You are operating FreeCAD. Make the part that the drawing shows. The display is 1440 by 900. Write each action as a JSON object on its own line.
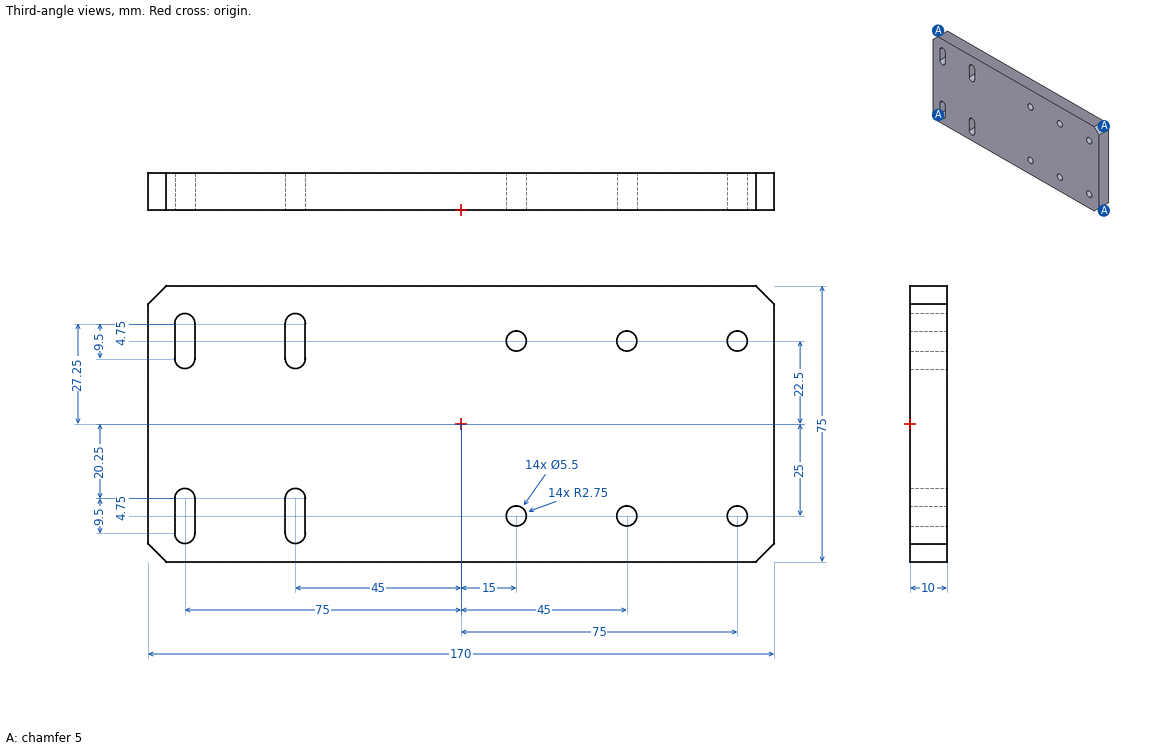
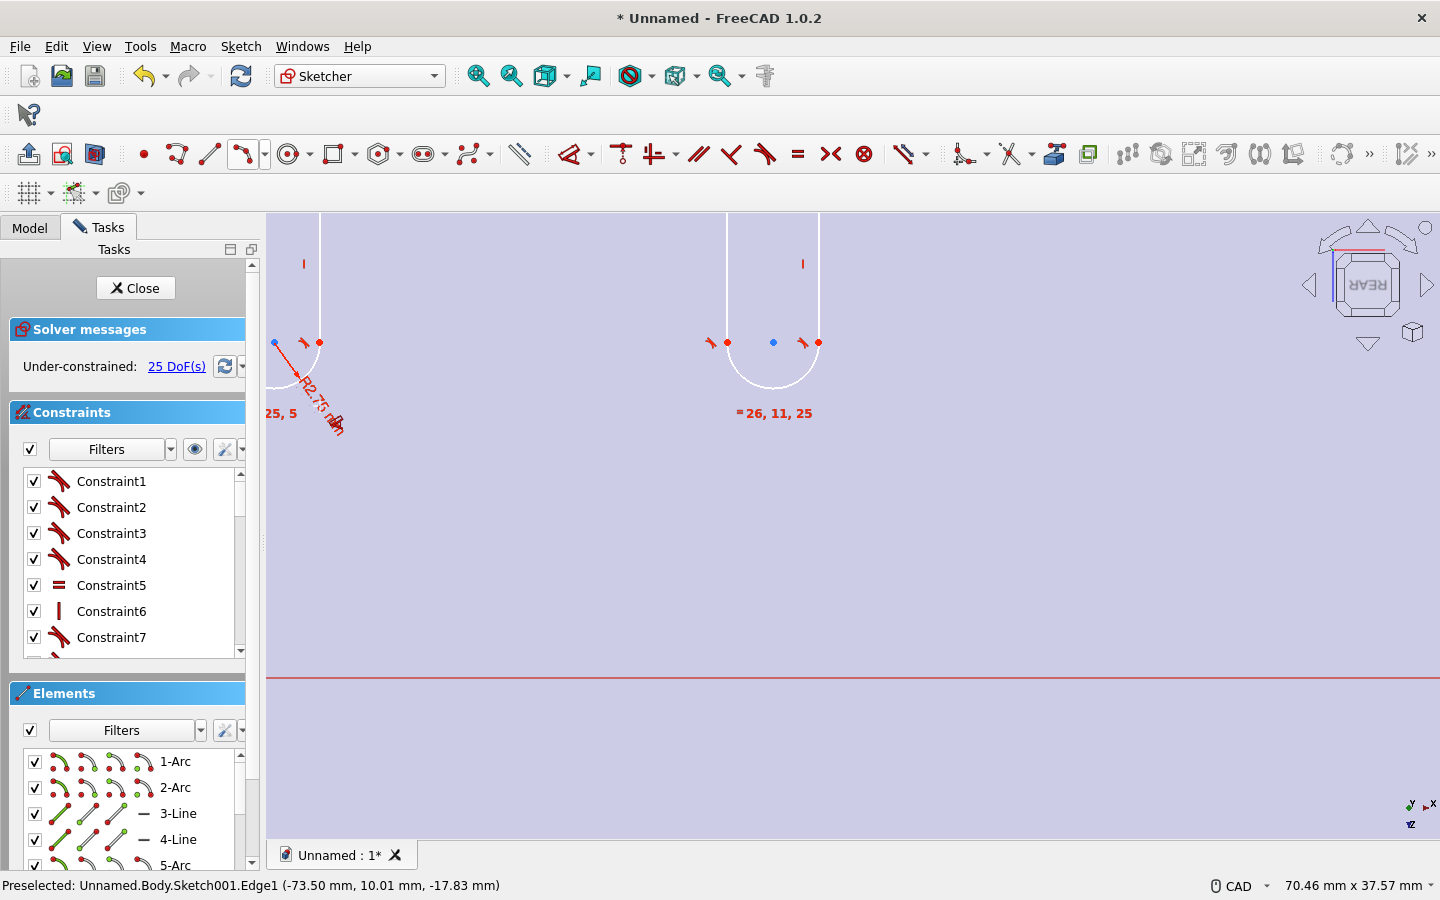
{"action": "scroll", "coordinate": [543, 483], "scroll_direction": "down", "scroll_amount": 7}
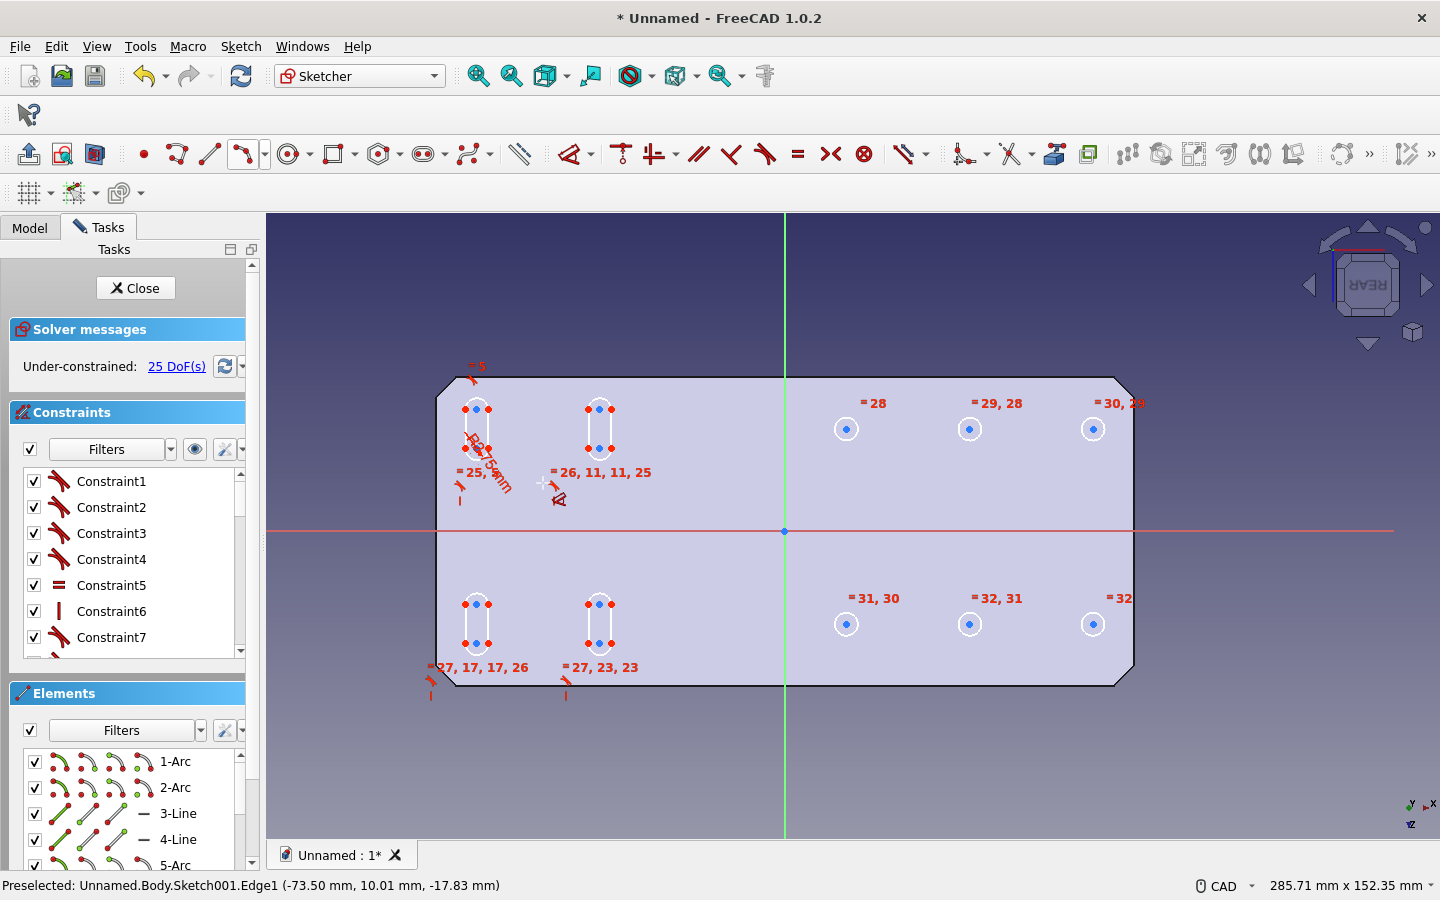
{"action": "scroll", "coordinate": [854, 421], "scroll_direction": "up", "scroll_amount": 3}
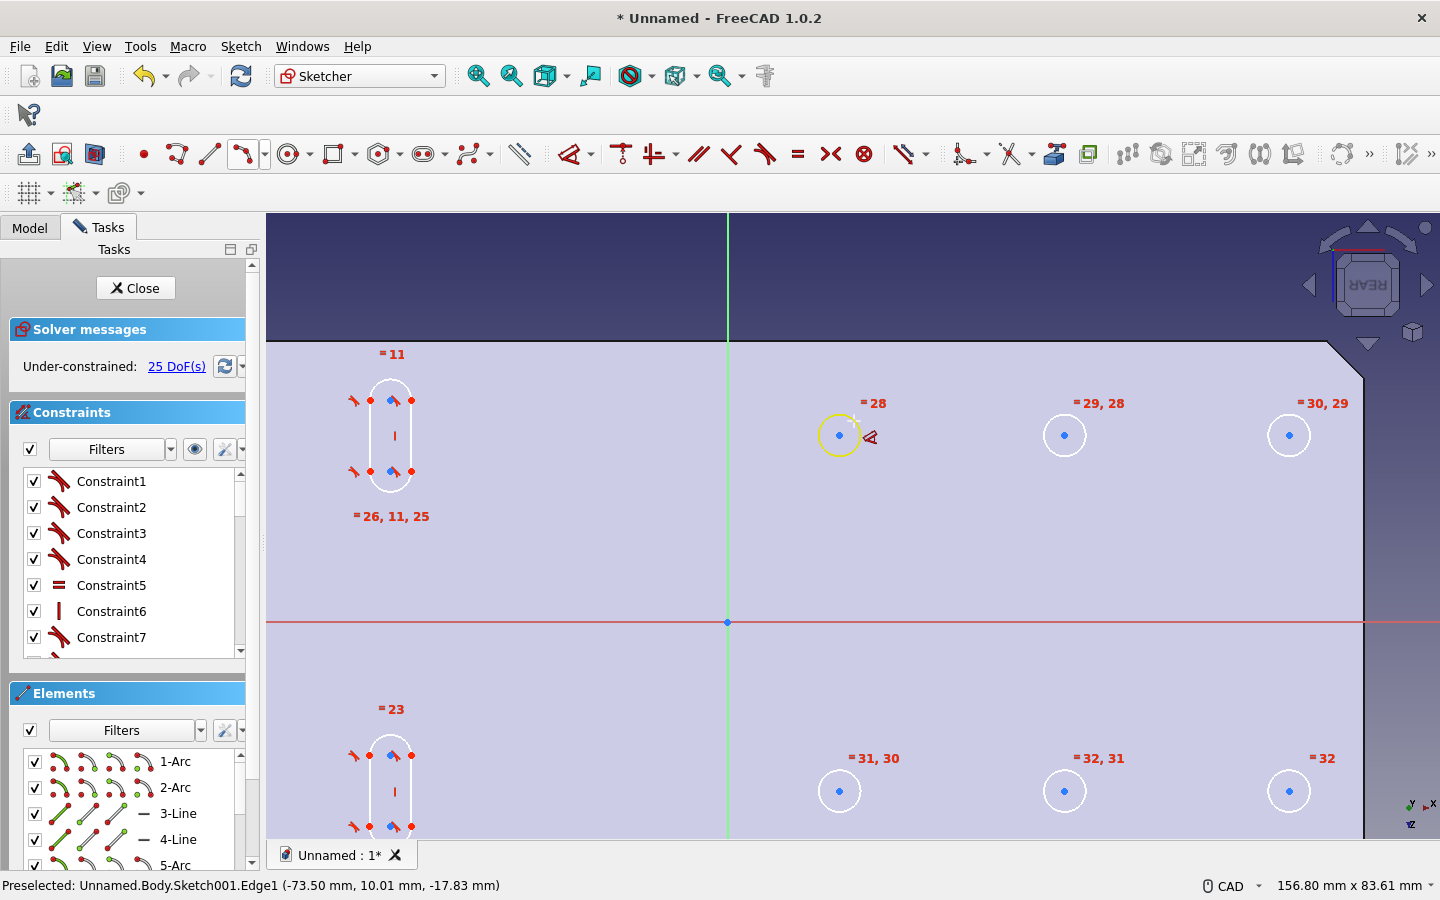
{"action": "left_click", "coordinate": [854, 421]}
{"action": "left_click", "coordinate": [877, 398]}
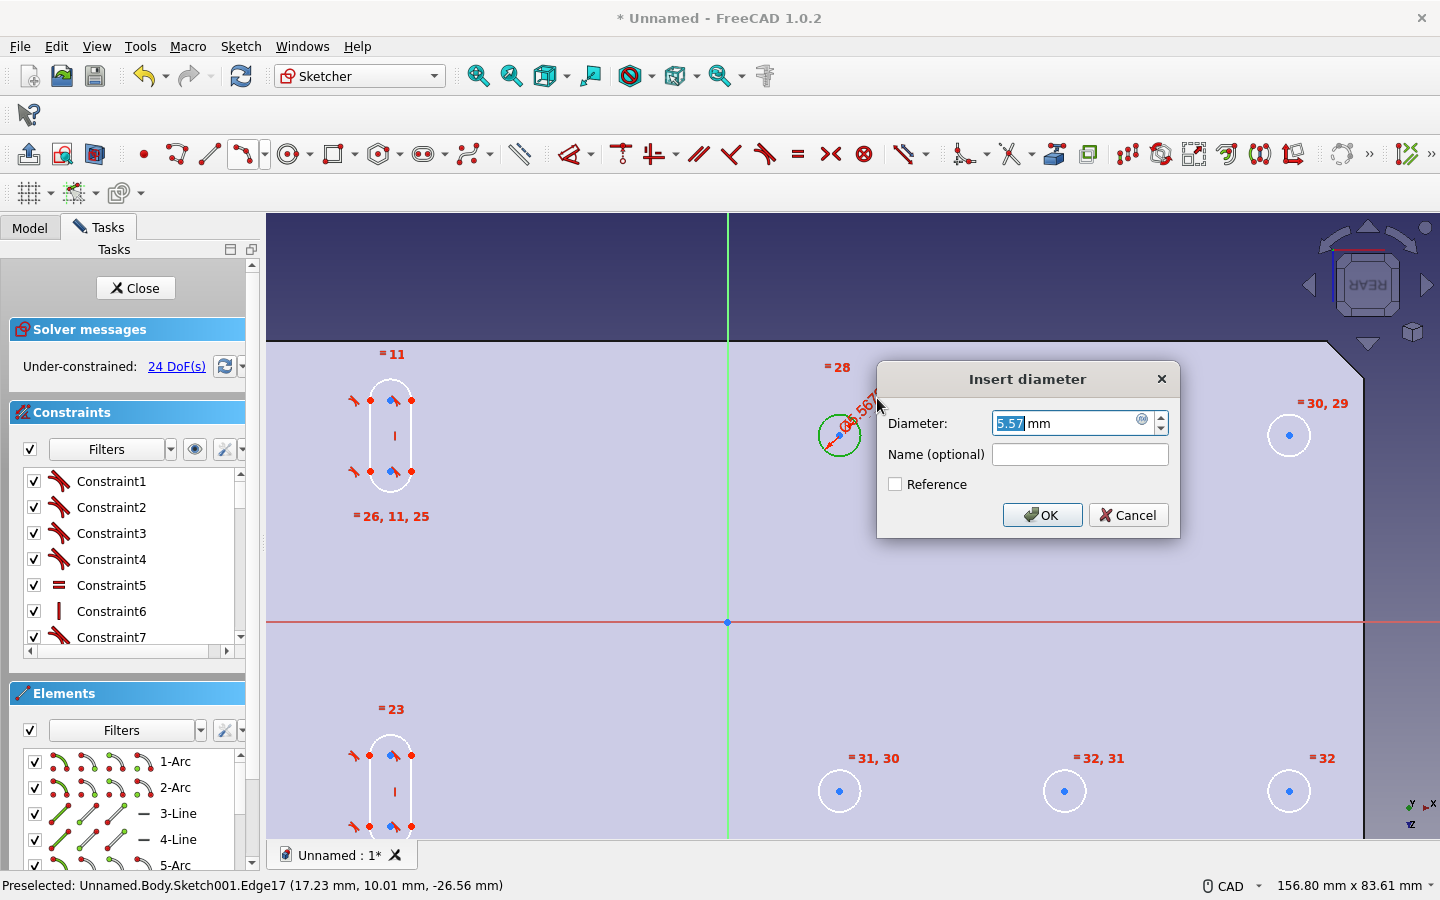
{"action": "type", "text": "5.5"}
{"action": "key", "text": "Return"}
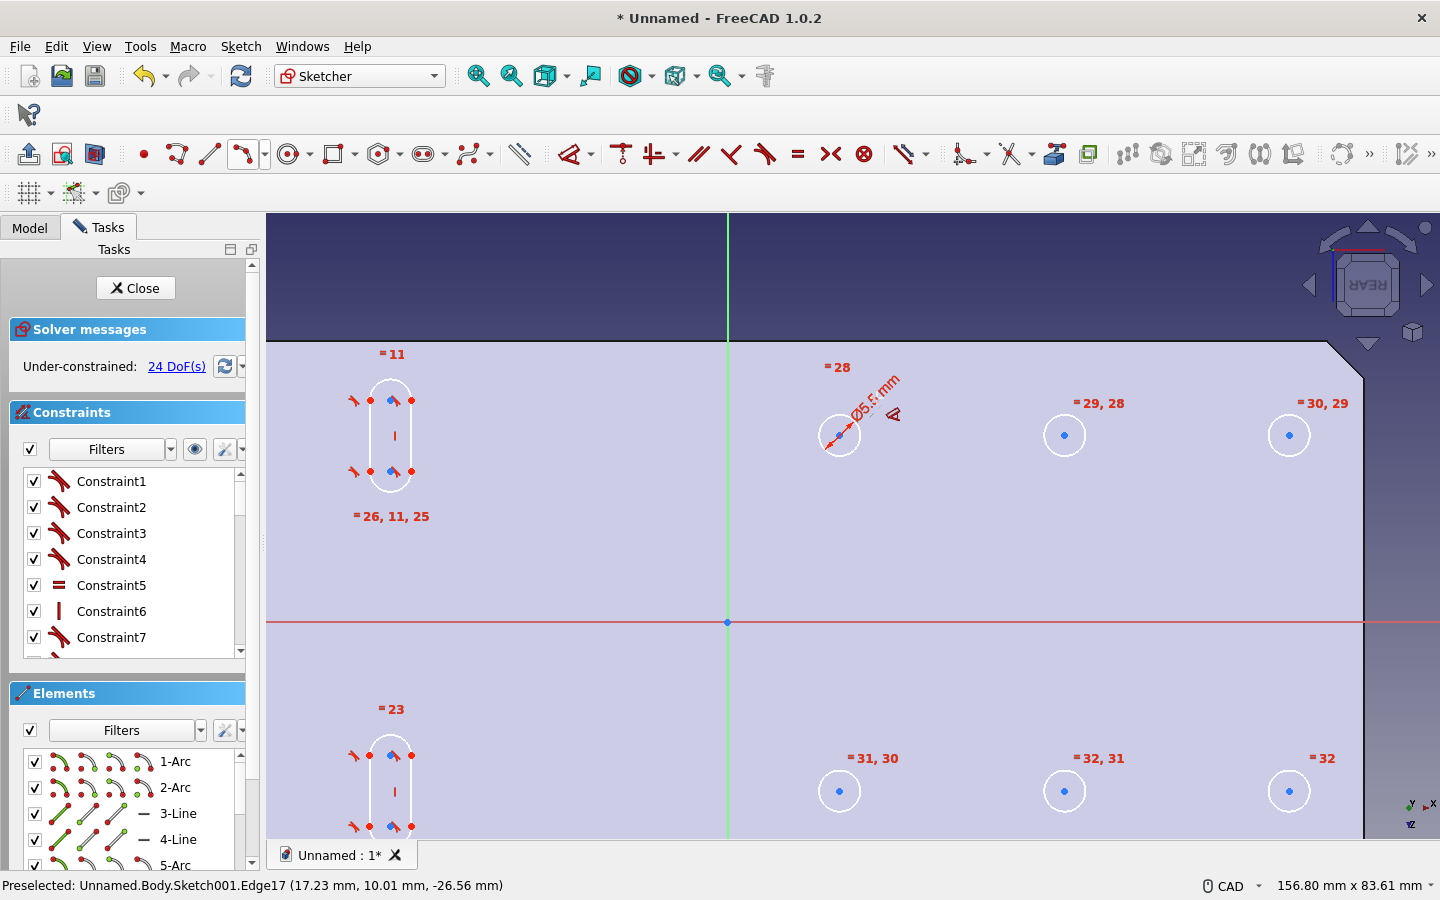
{"action": "left_click", "coordinate": [840, 435]}
{"action": "left_click", "coordinate": [784, 401]}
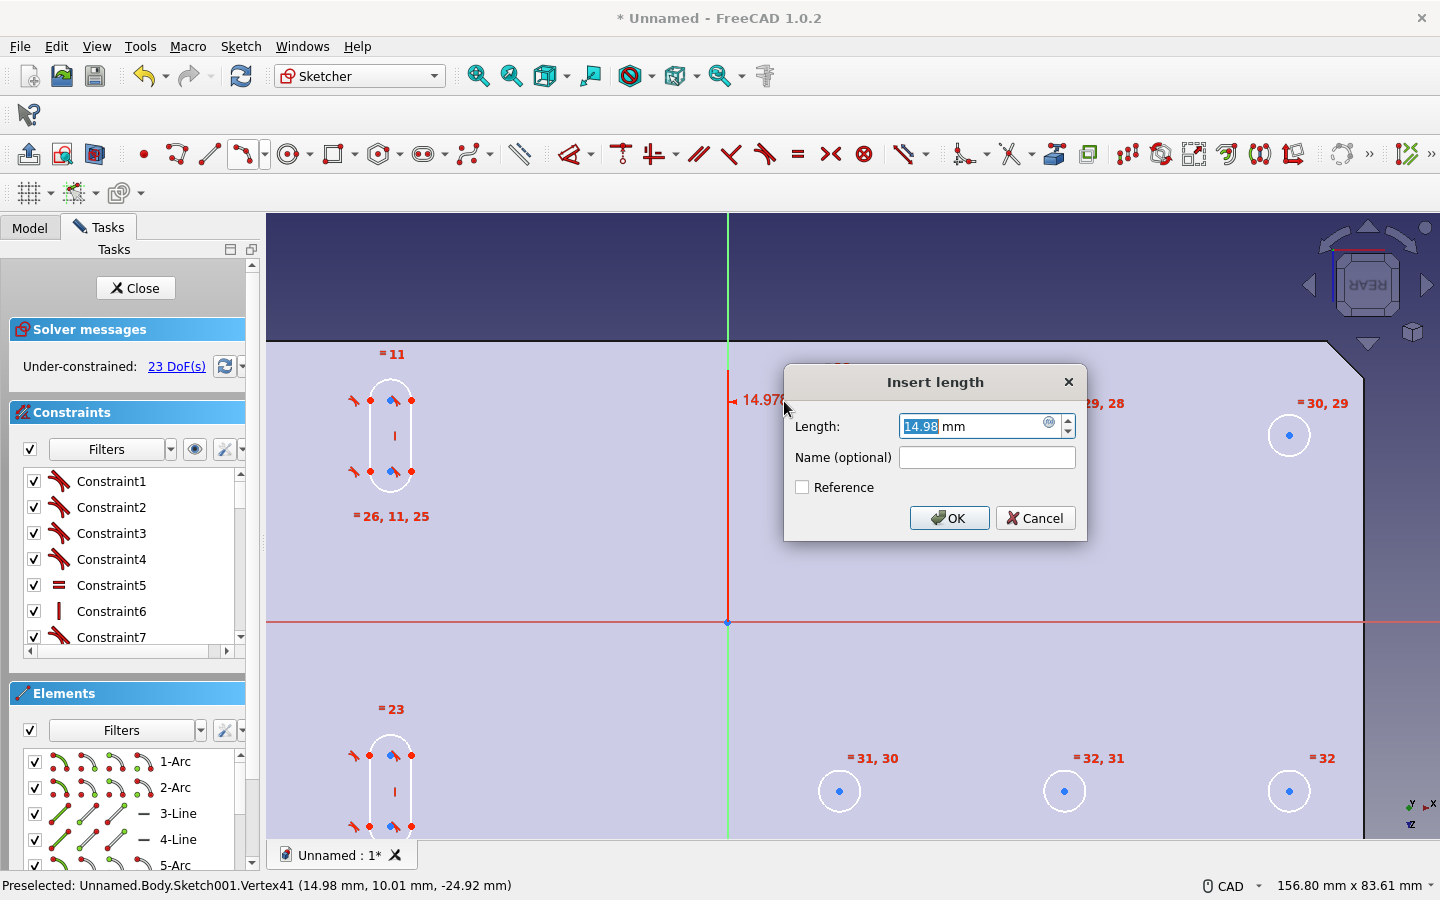
{"action": "type", "text": "15"}
{"action": "key", "text": "Return"}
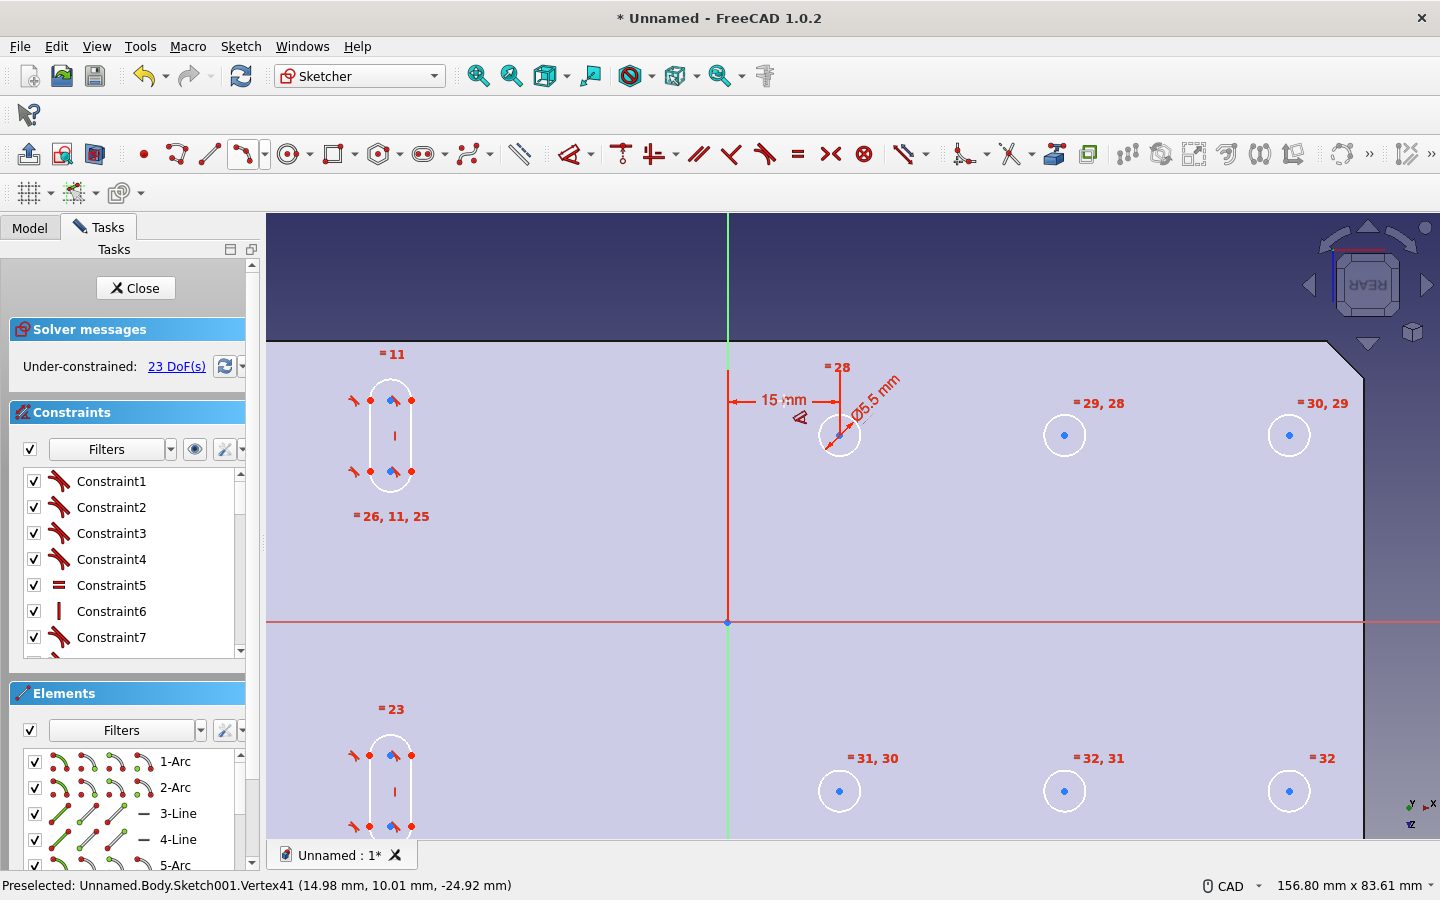
{"action": "left_click", "coordinate": [840, 435]}
{"action": "left_click", "coordinate": [874, 529]}